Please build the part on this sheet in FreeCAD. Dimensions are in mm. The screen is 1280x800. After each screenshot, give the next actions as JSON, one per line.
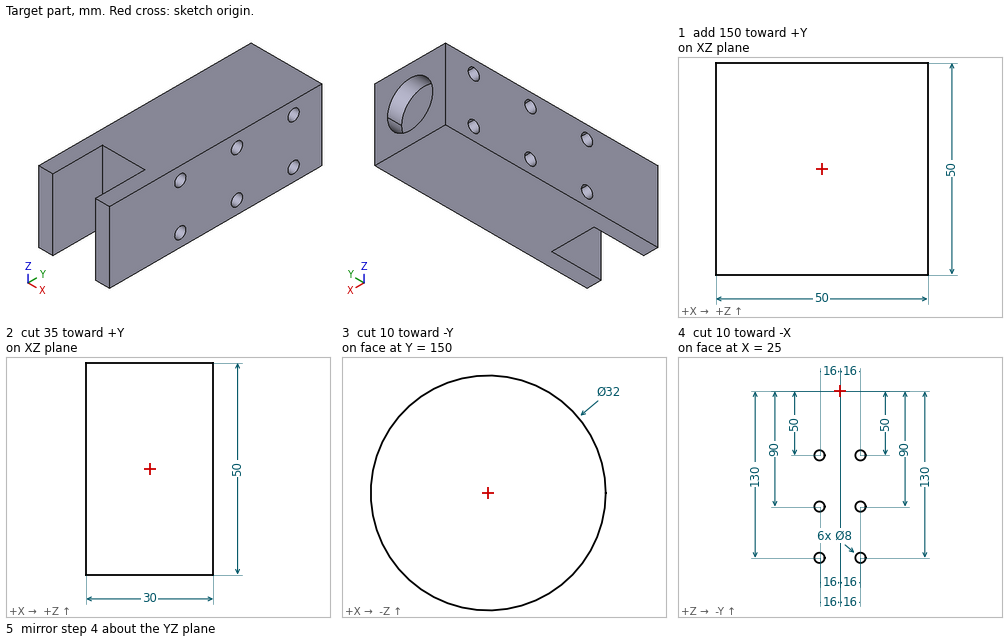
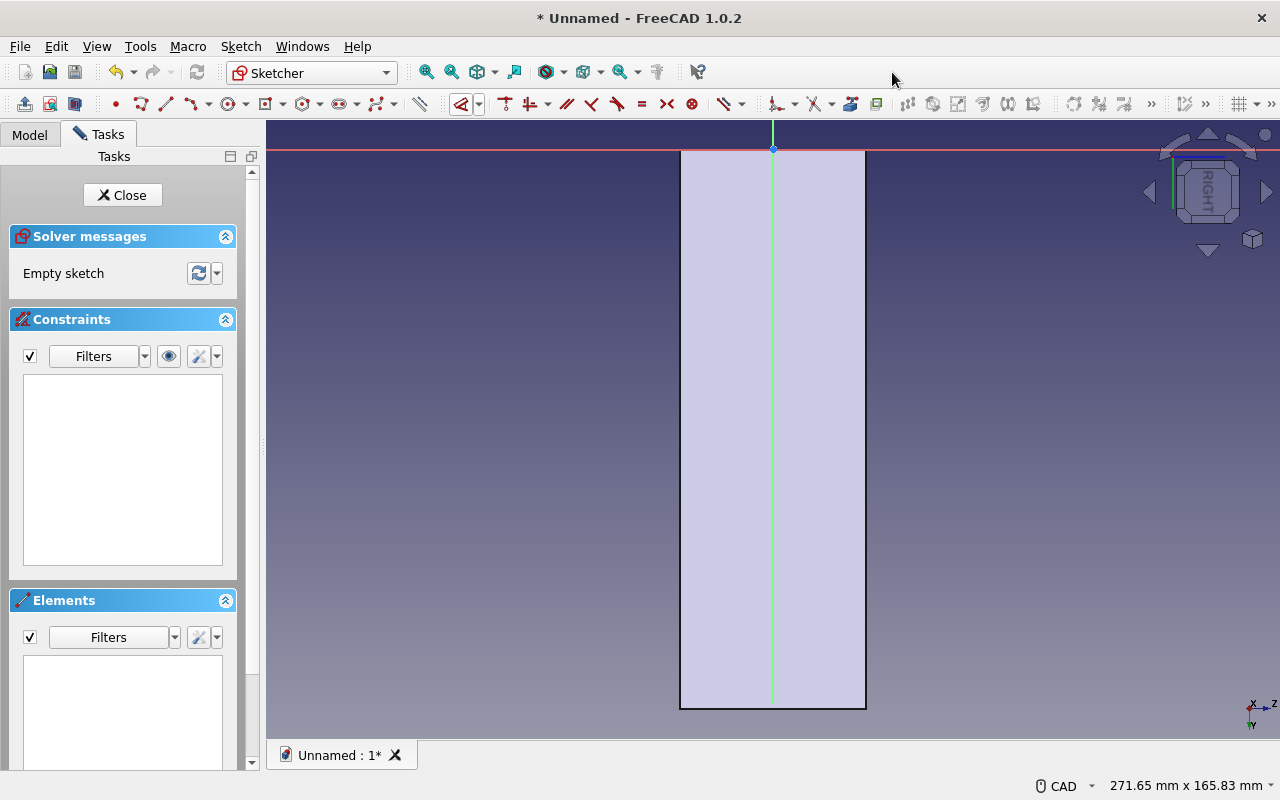
{"action": "scroll", "coordinate": [395, 564], "scroll_direction": "down", "scroll_amount": 1}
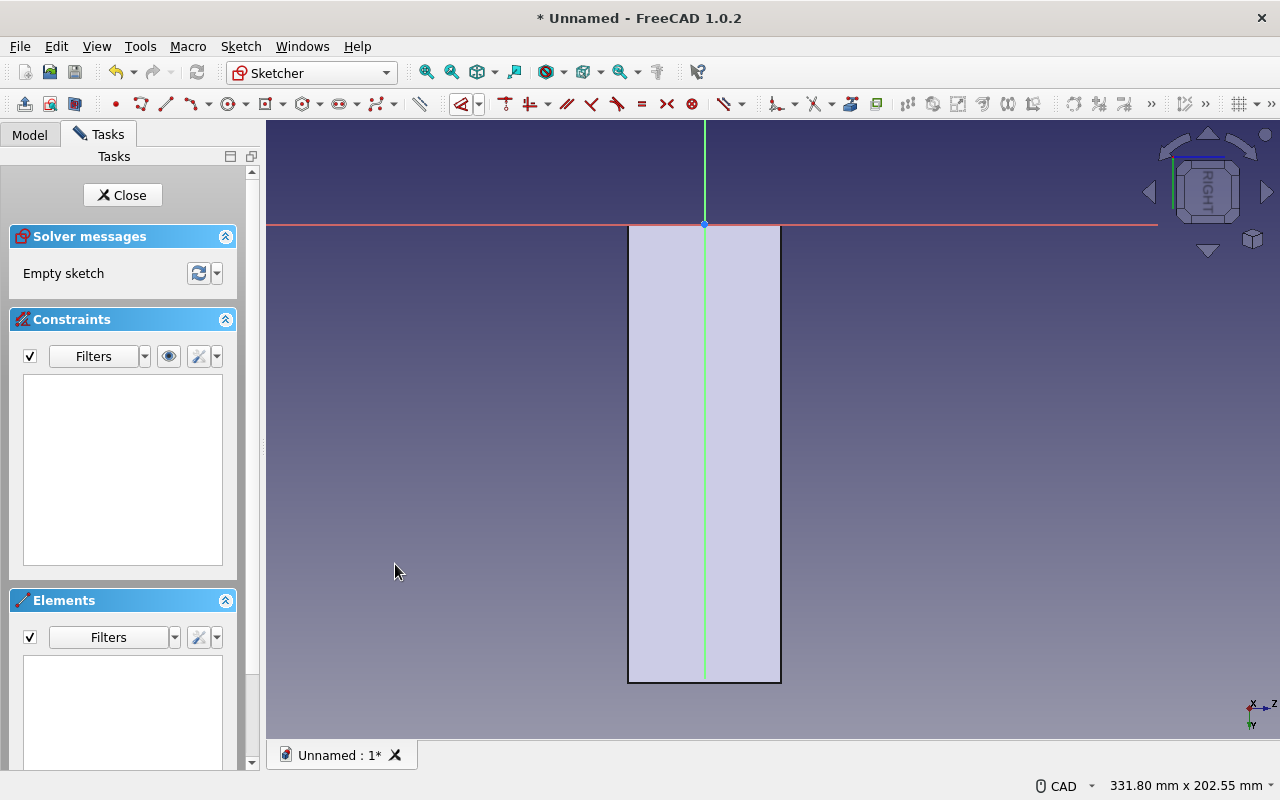
{"action": "left_click", "coordinate": [228, 104]}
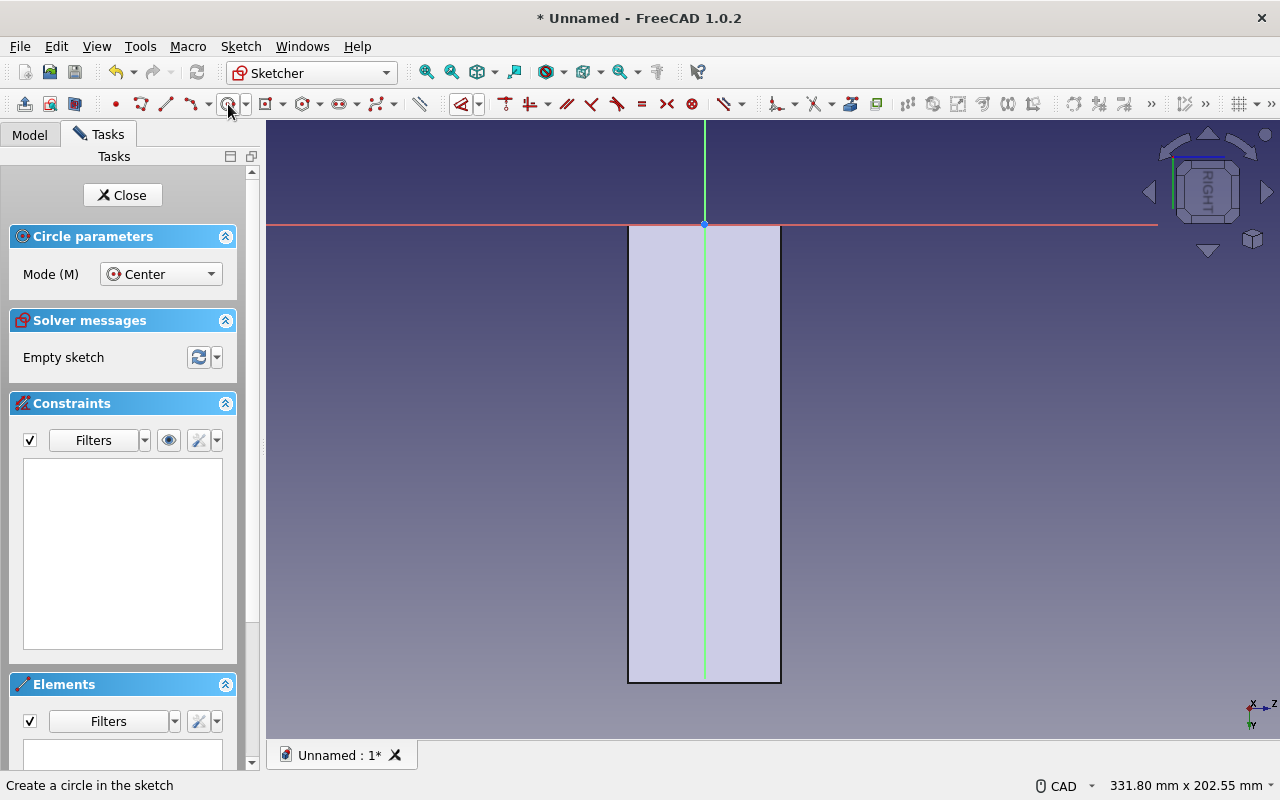
{"action": "scroll", "coordinate": [753, 622], "scroll_direction": "up", "scroll_amount": 4}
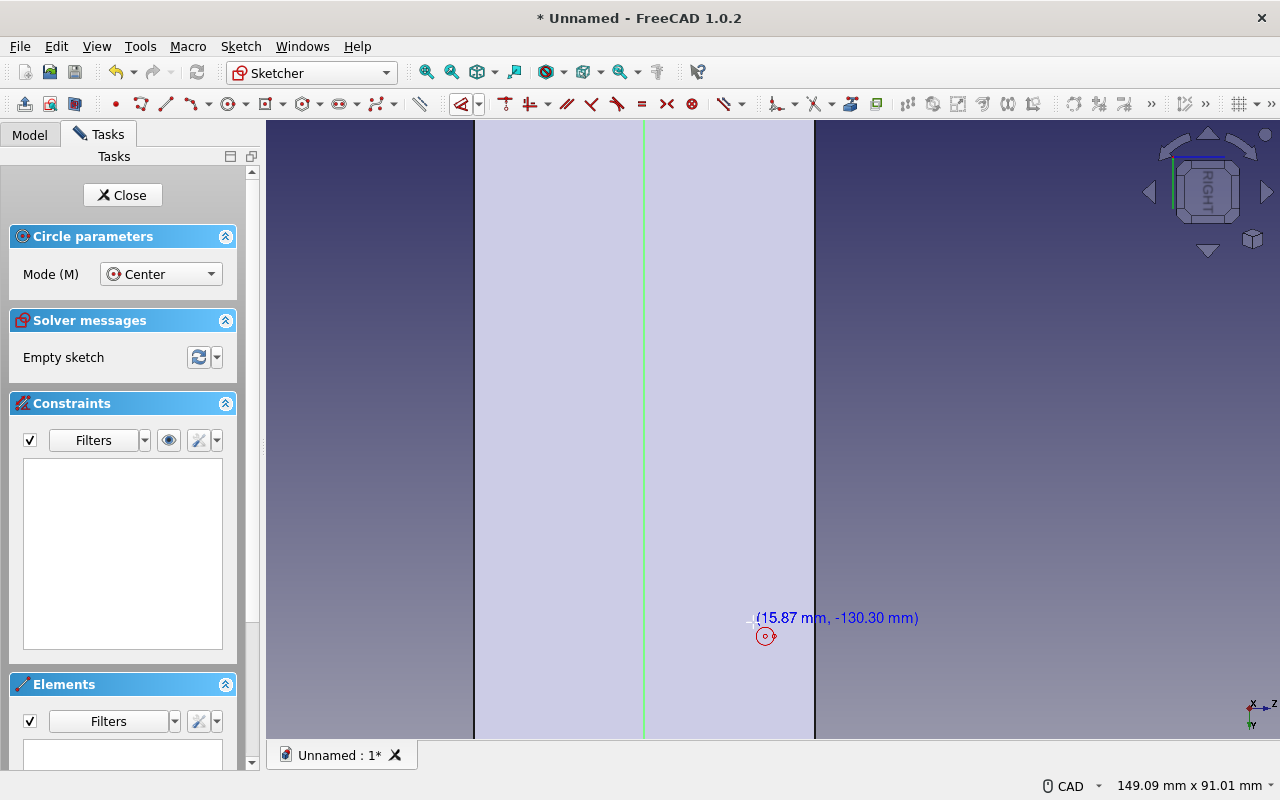
{"action": "left_click", "coordinate": [753, 621]}
{"action": "mouse_move", "coordinate": [773, 602]}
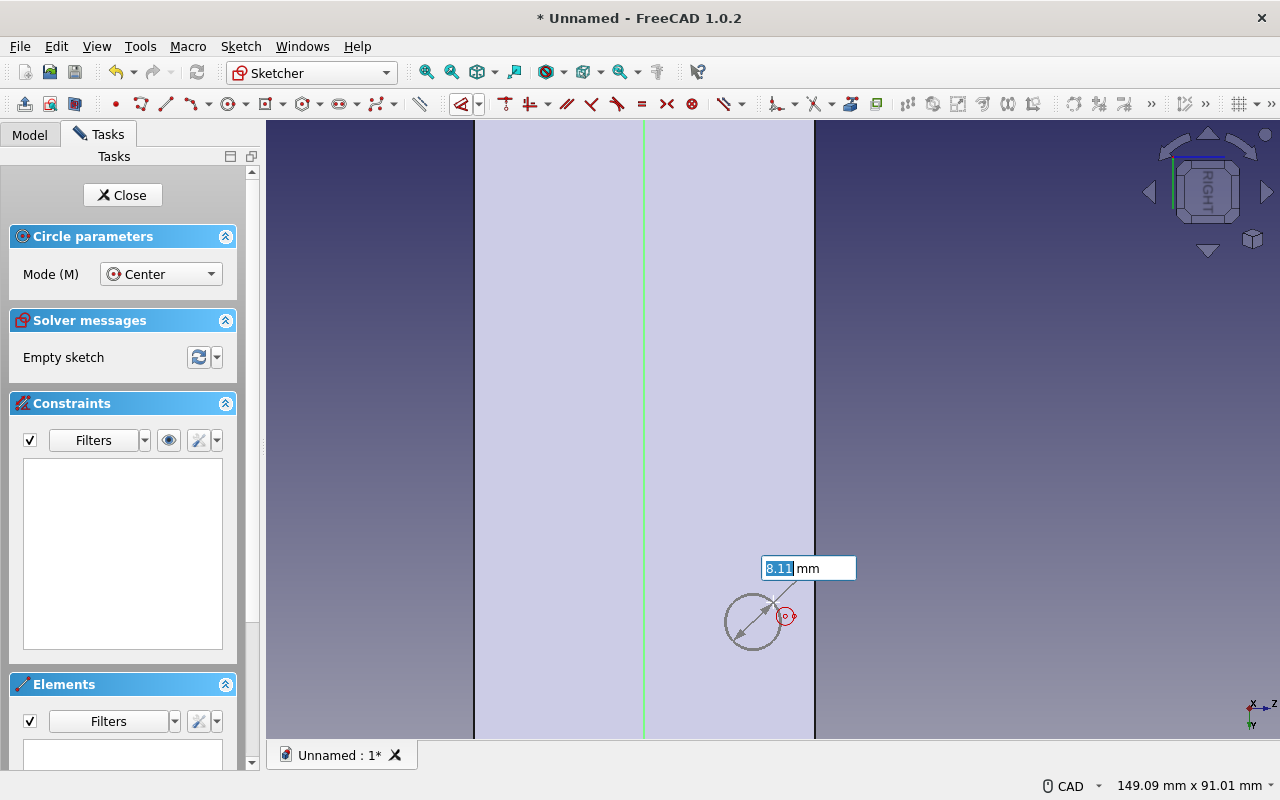
{"action": "type", "text": "8"}
{"action": "key", "text": "Return"}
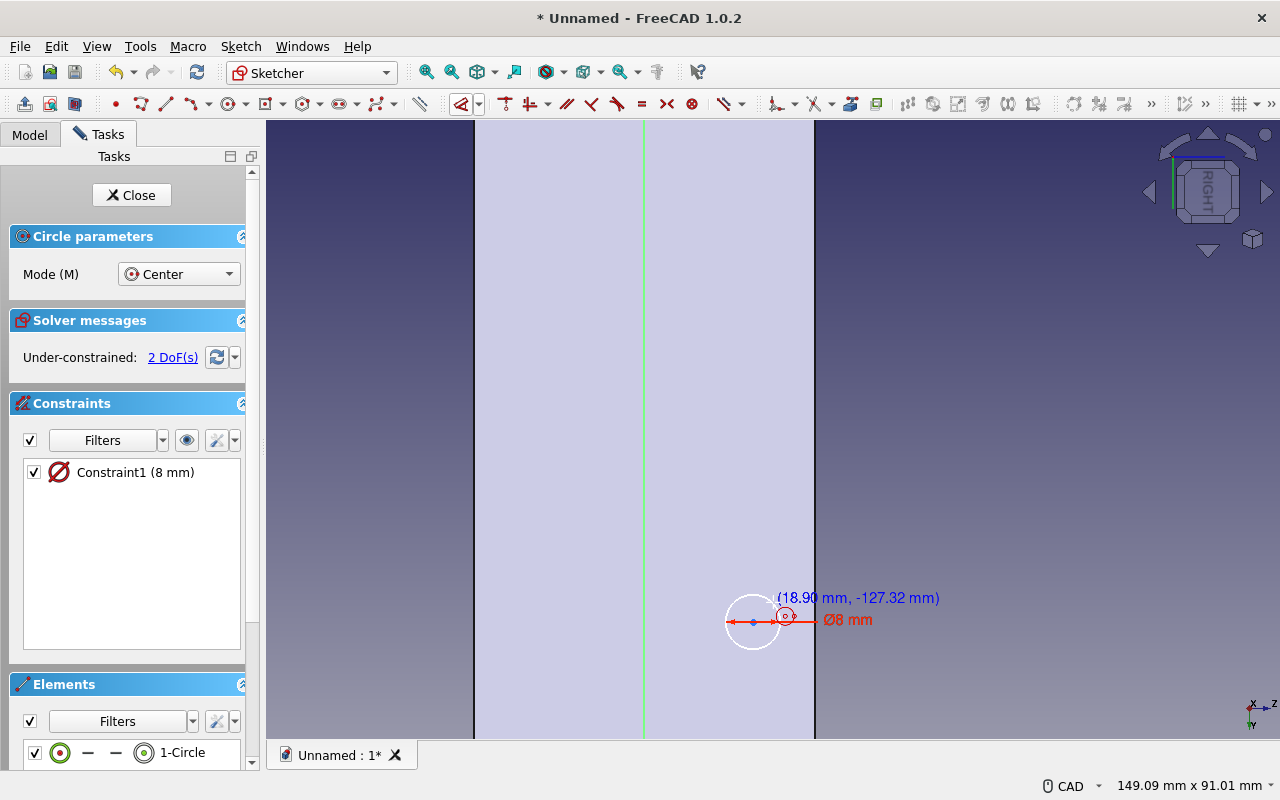
{"action": "left_click", "coordinate": [536, 621]}
{"action": "mouse_move", "coordinate": [555, 602]}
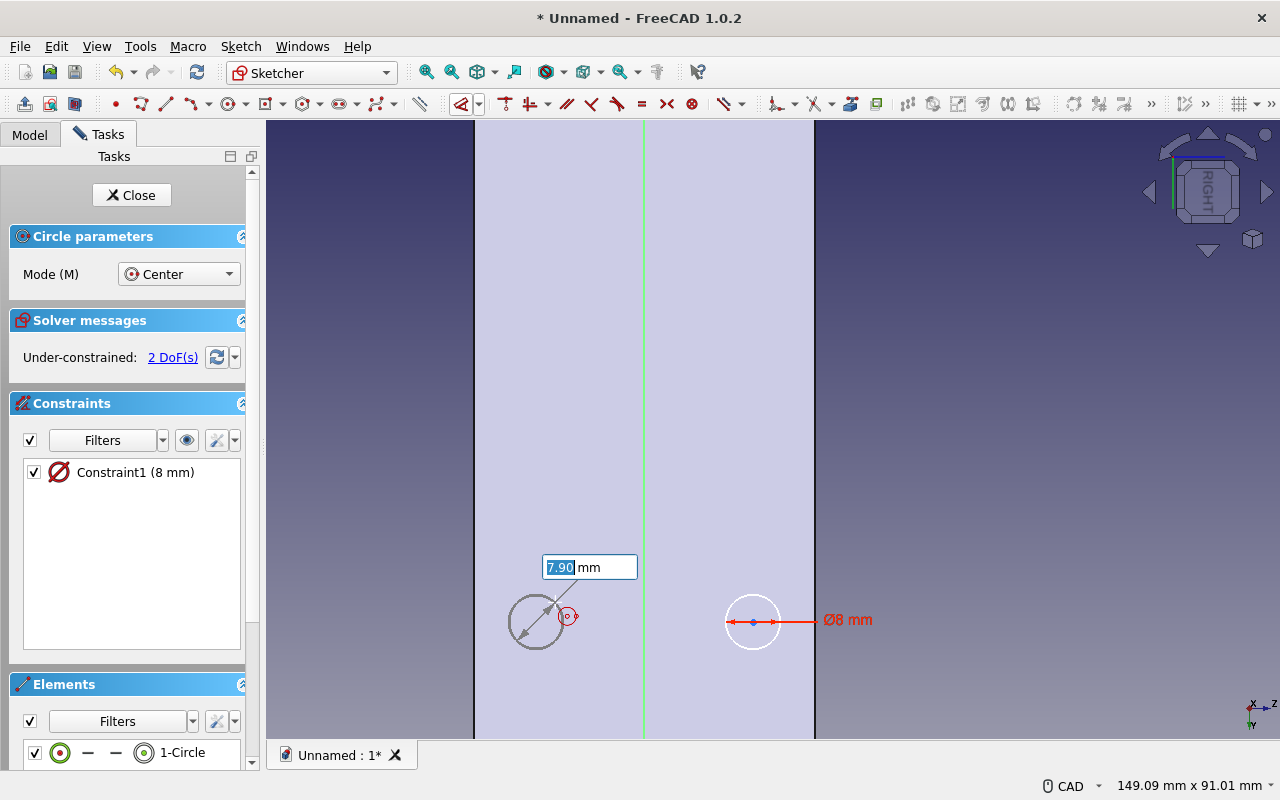
{"action": "type", "text": "8"}
{"action": "key", "text": "Return"}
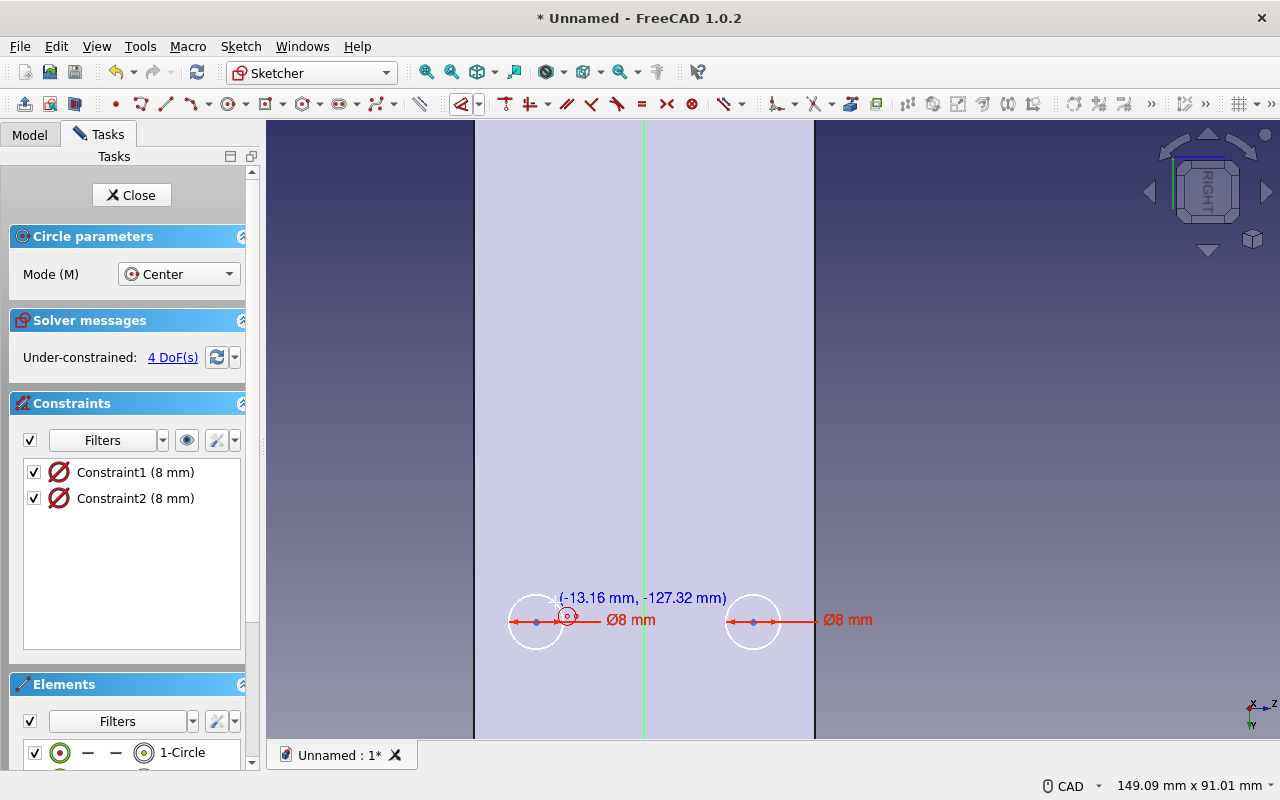
{"action": "left_click", "coordinate": [753, 349]}
{"action": "mouse_move", "coordinate": [773, 330]}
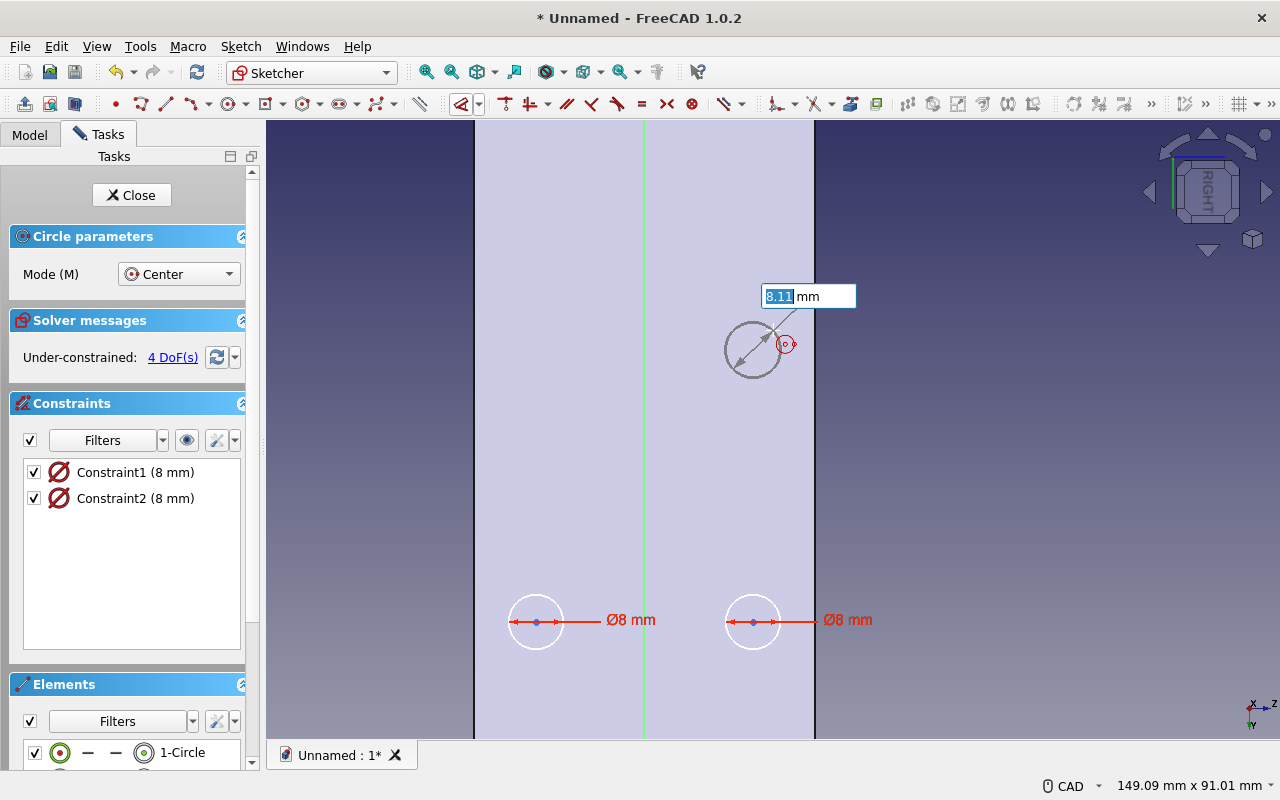
{"action": "type", "text": "8"}
{"action": "key", "text": "Return"}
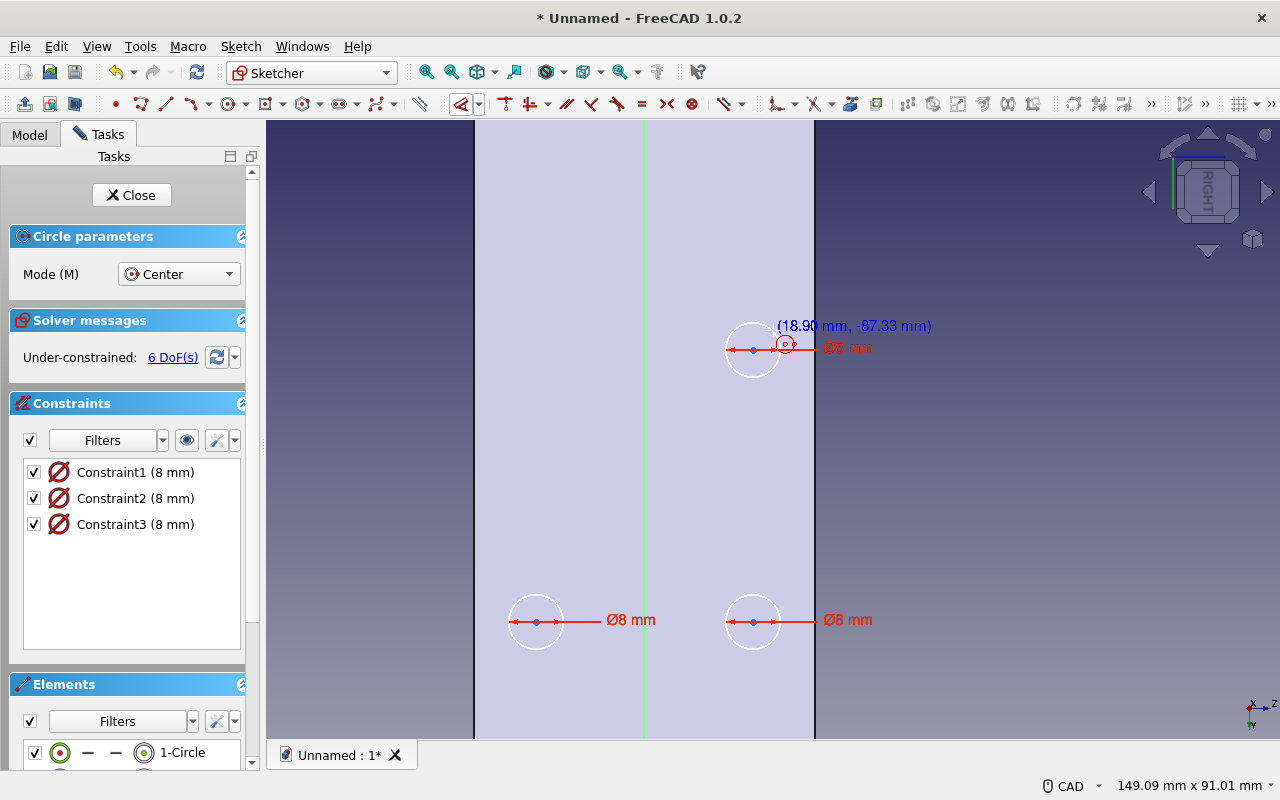
{"action": "scroll", "coordinate": [753, 623], "scroll_direction": "down", "scroll_amount": 4}